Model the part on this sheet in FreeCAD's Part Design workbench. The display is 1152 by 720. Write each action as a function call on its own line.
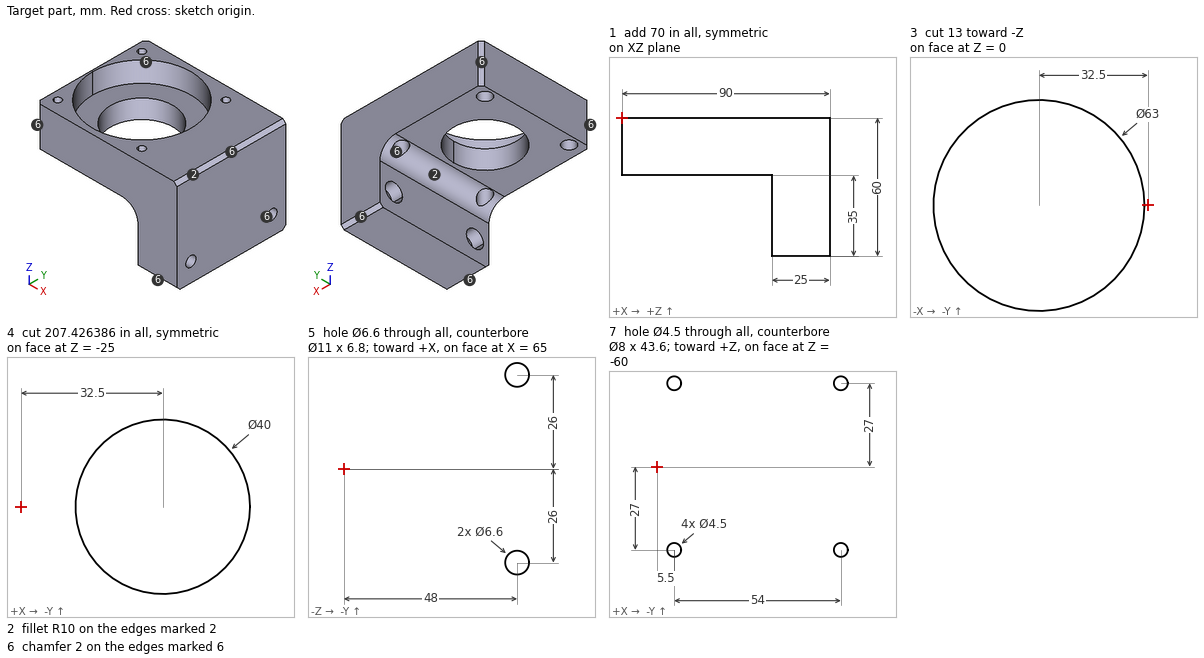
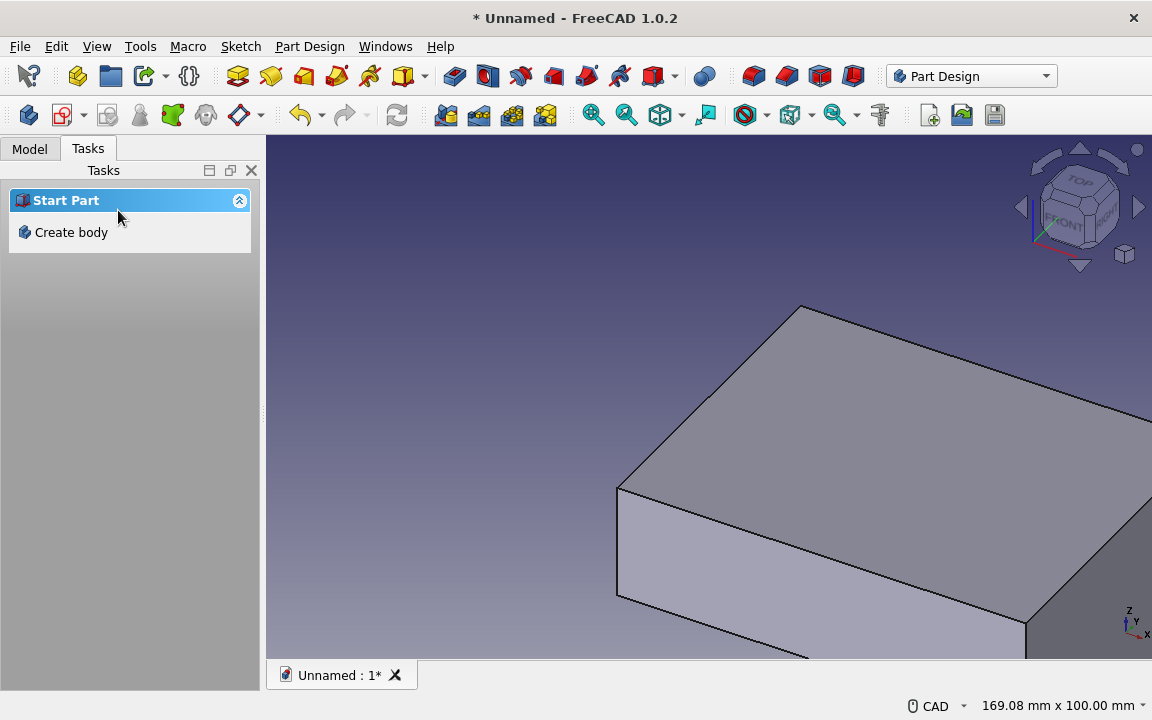
key(v)
key(f)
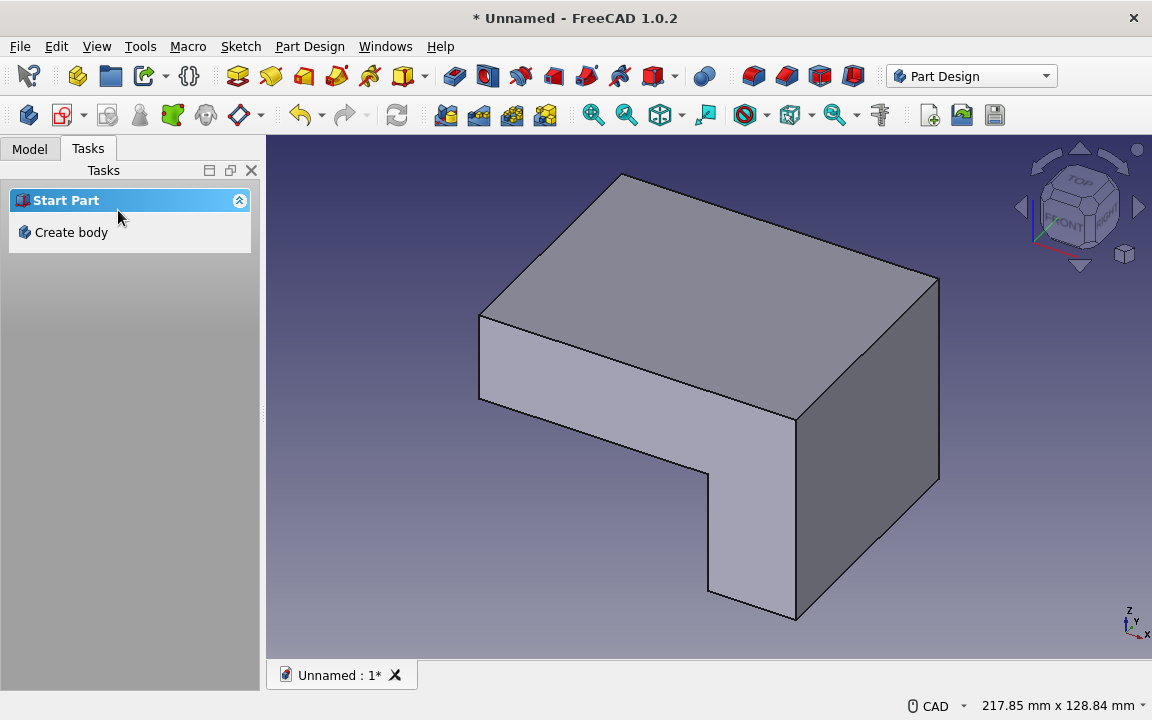
key(0)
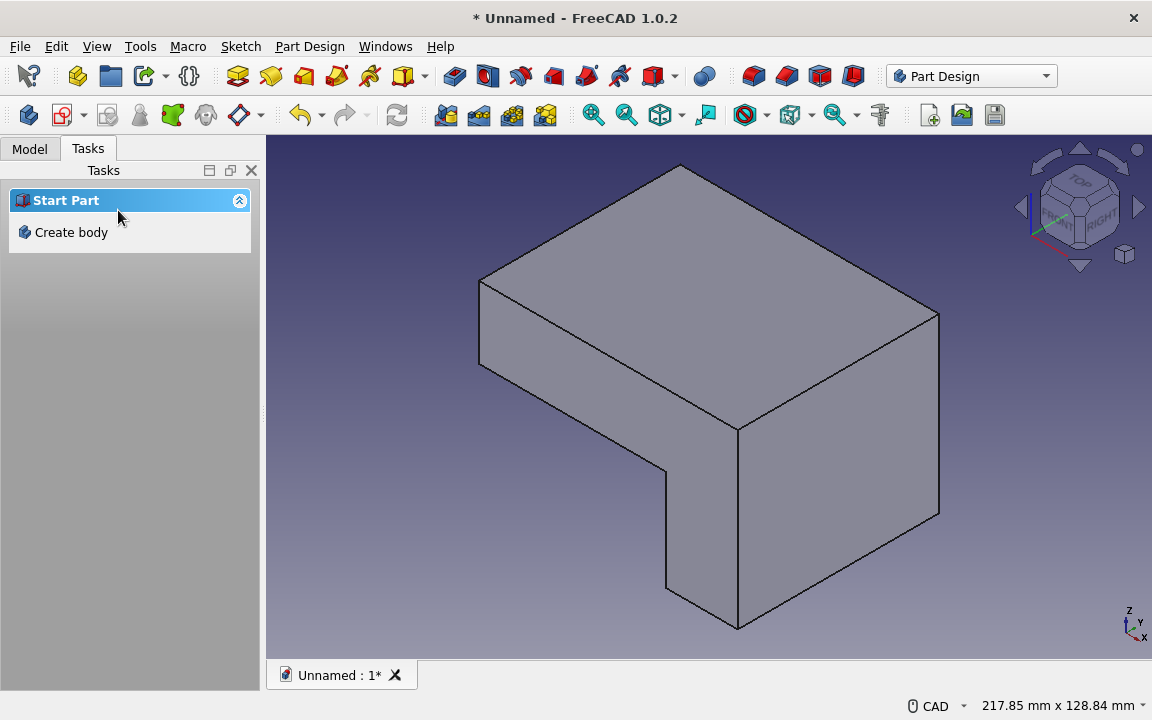
key(2)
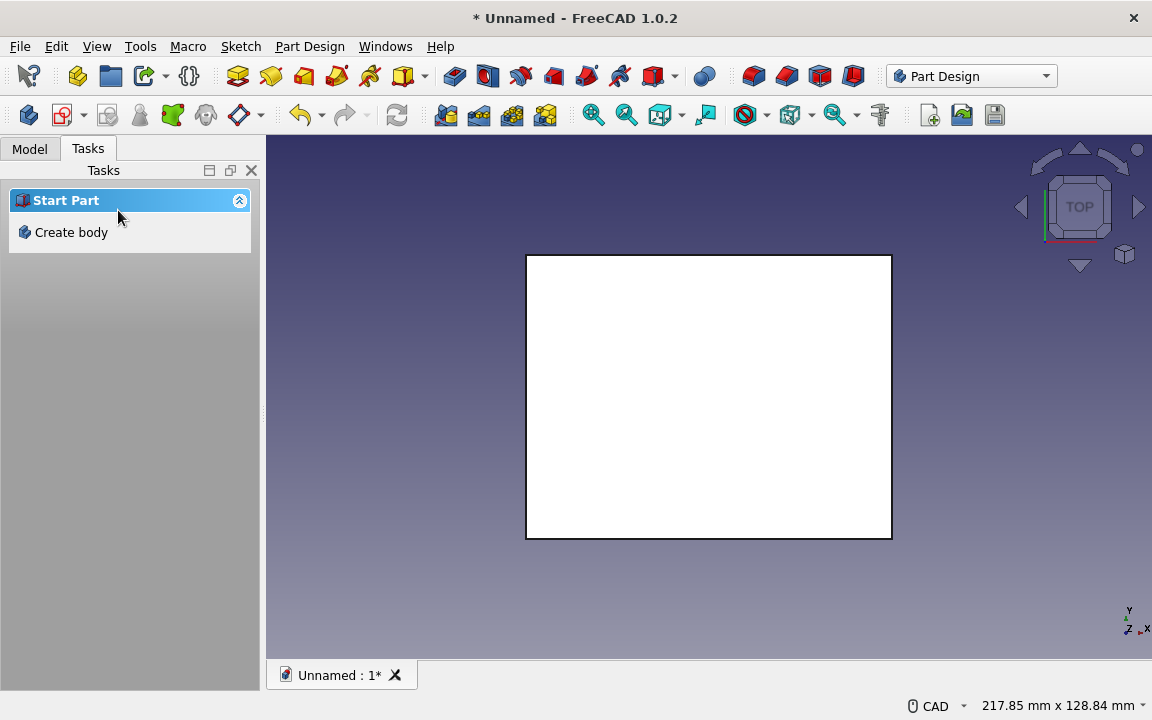
key(1)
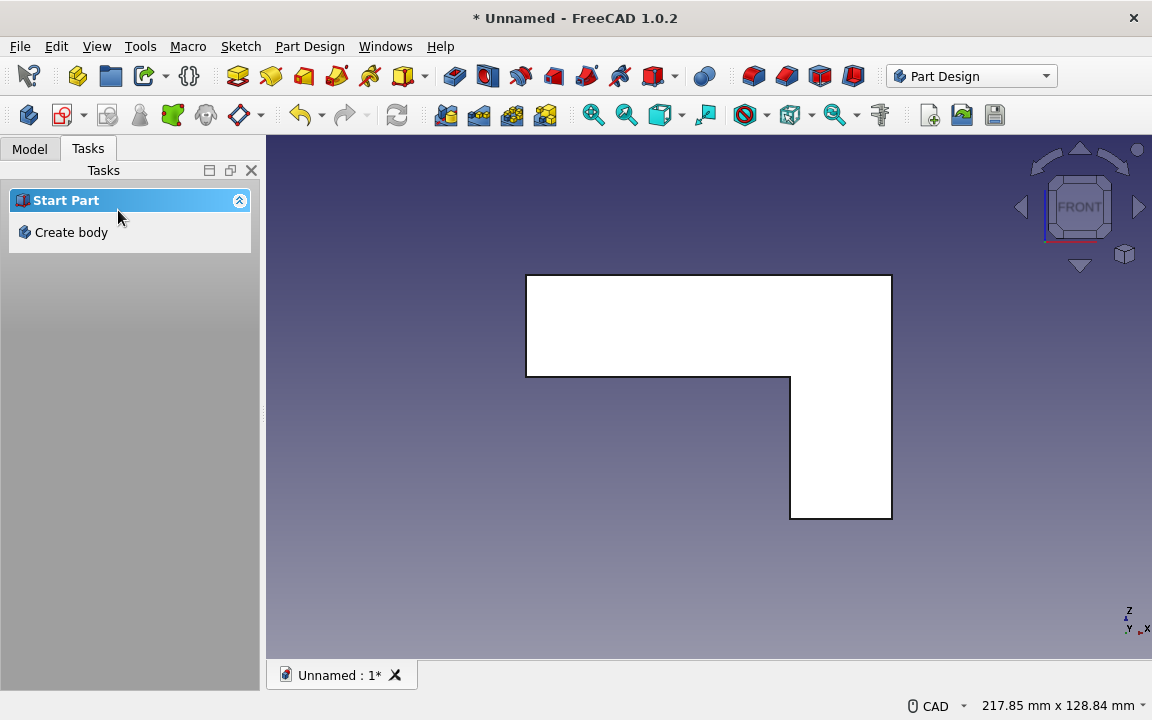
key(3)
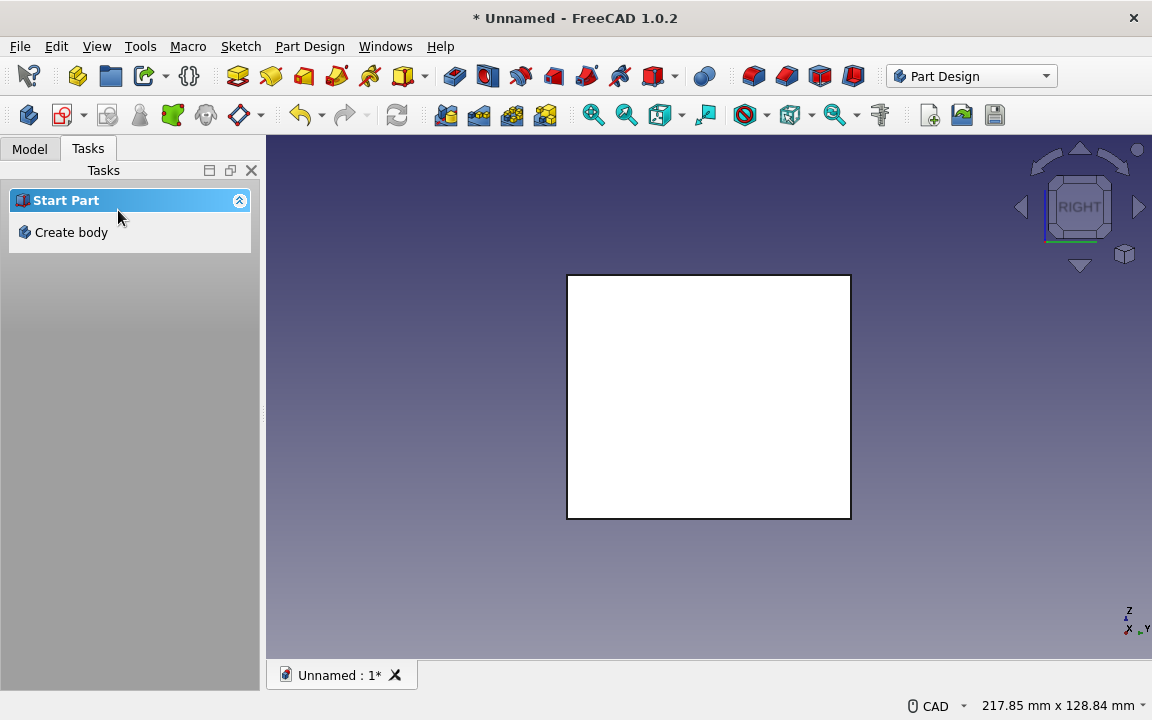
key(5)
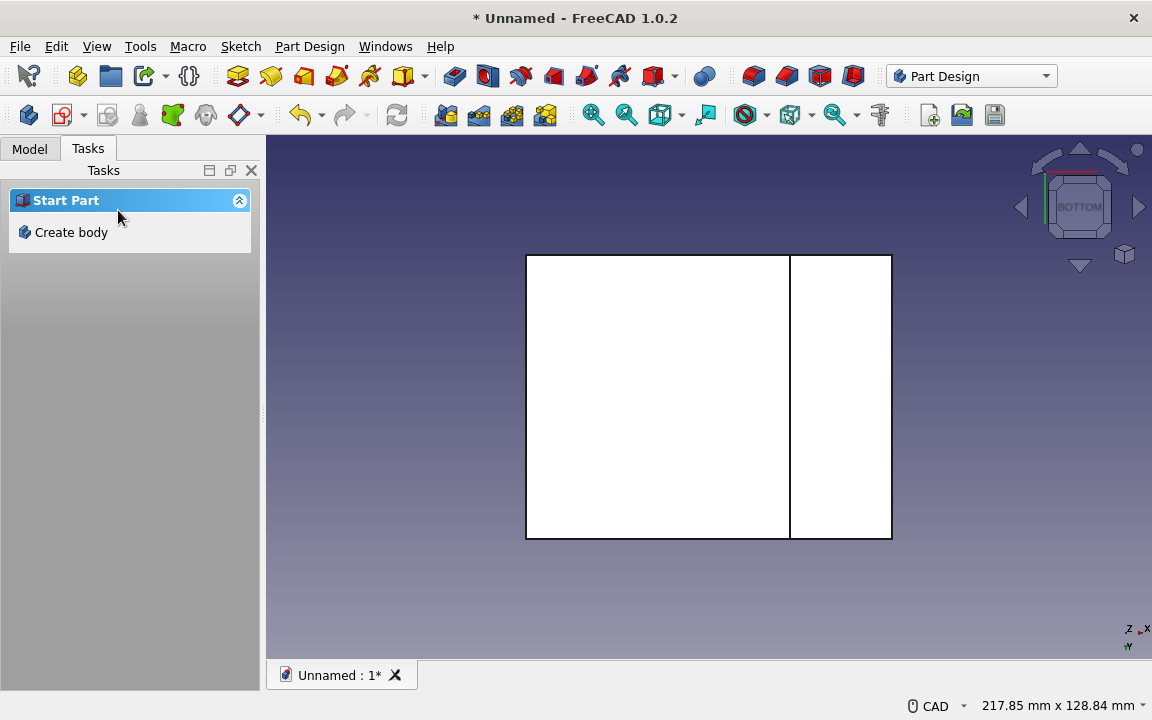
key(4)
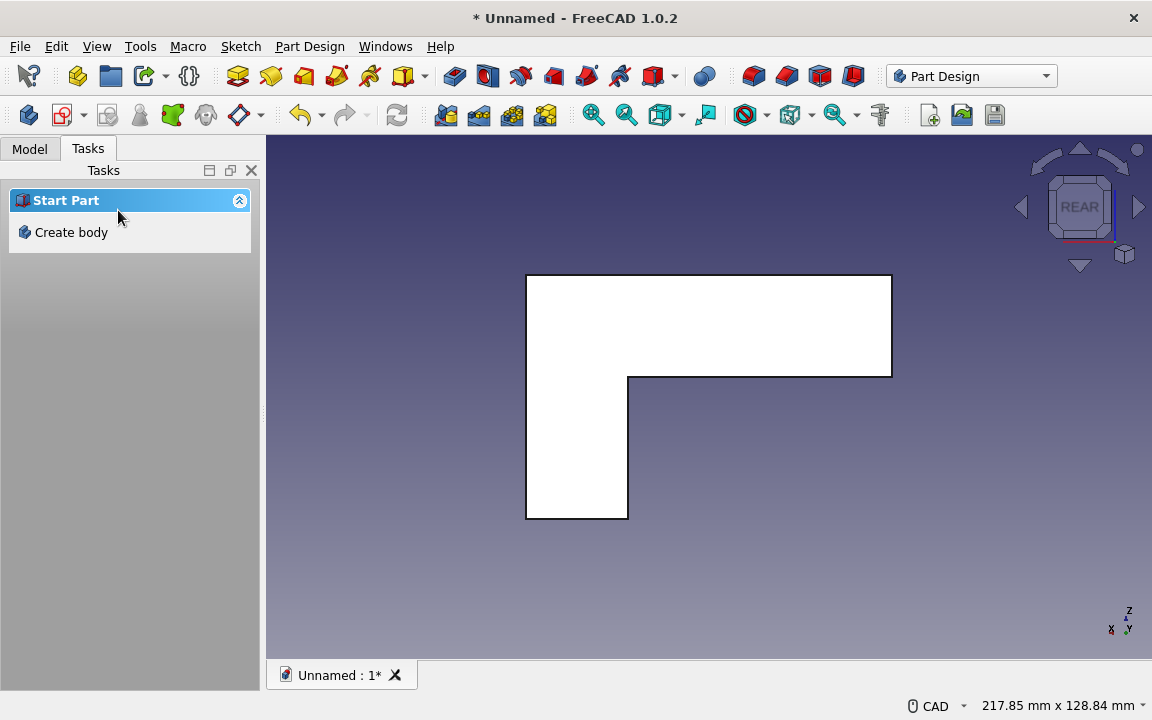
key(6)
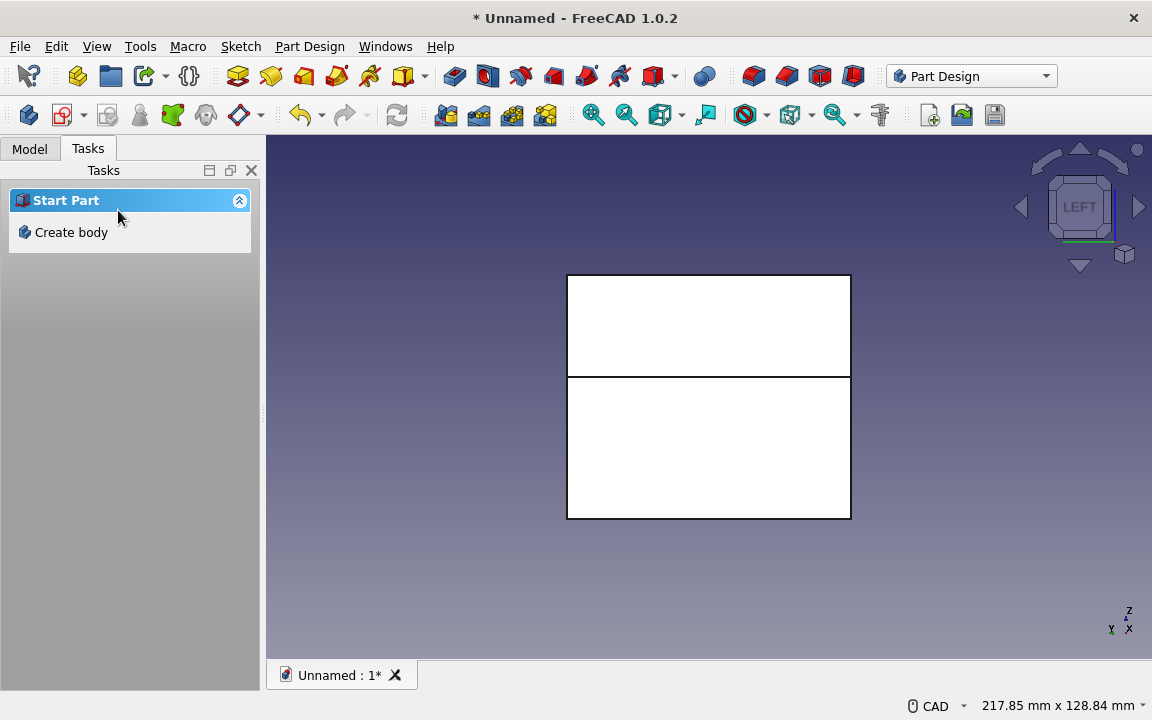
key(v)
key(3)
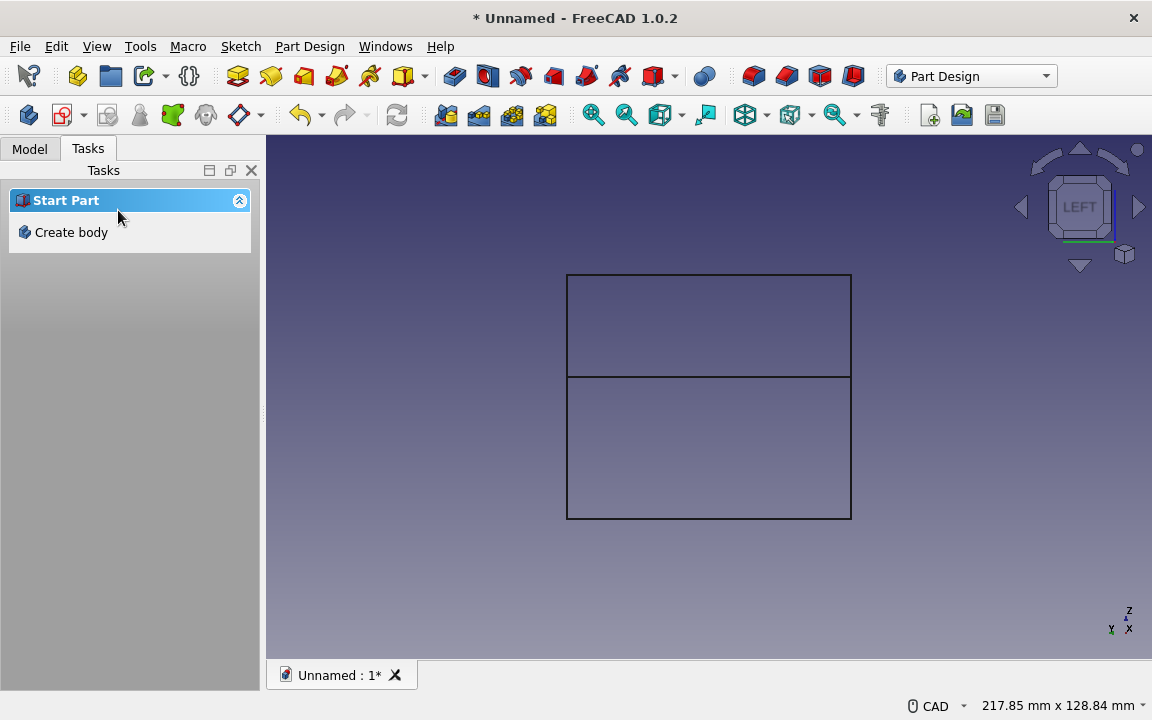
key(0)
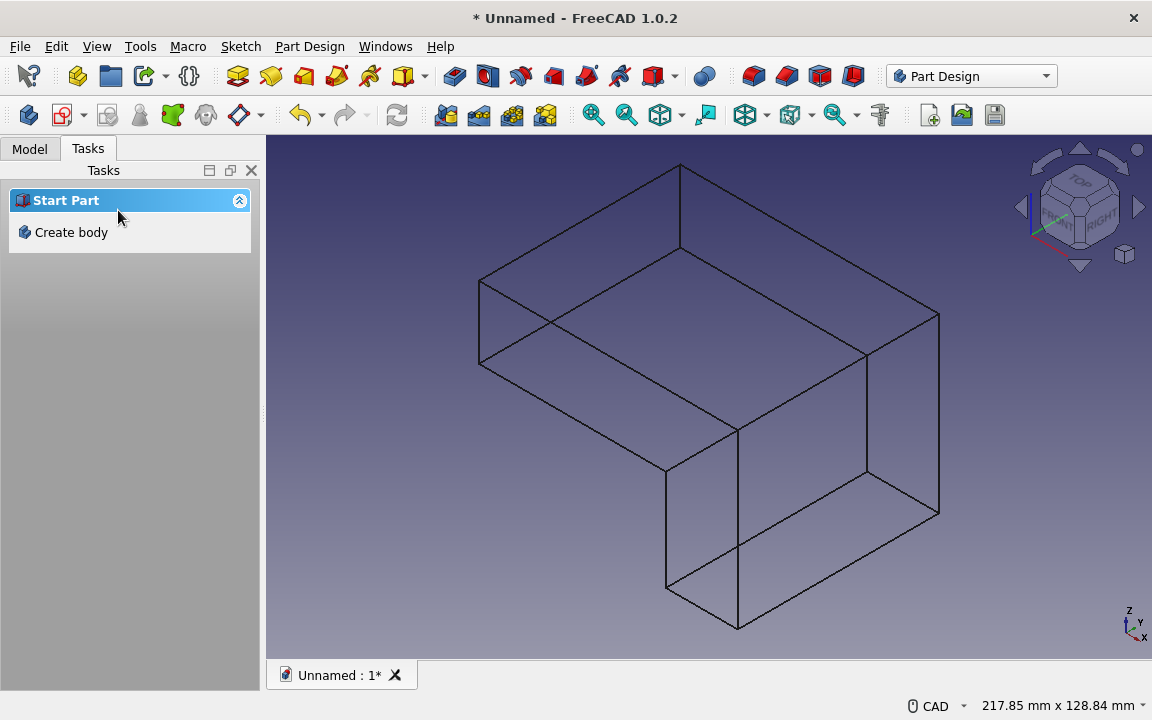
click(726, 436)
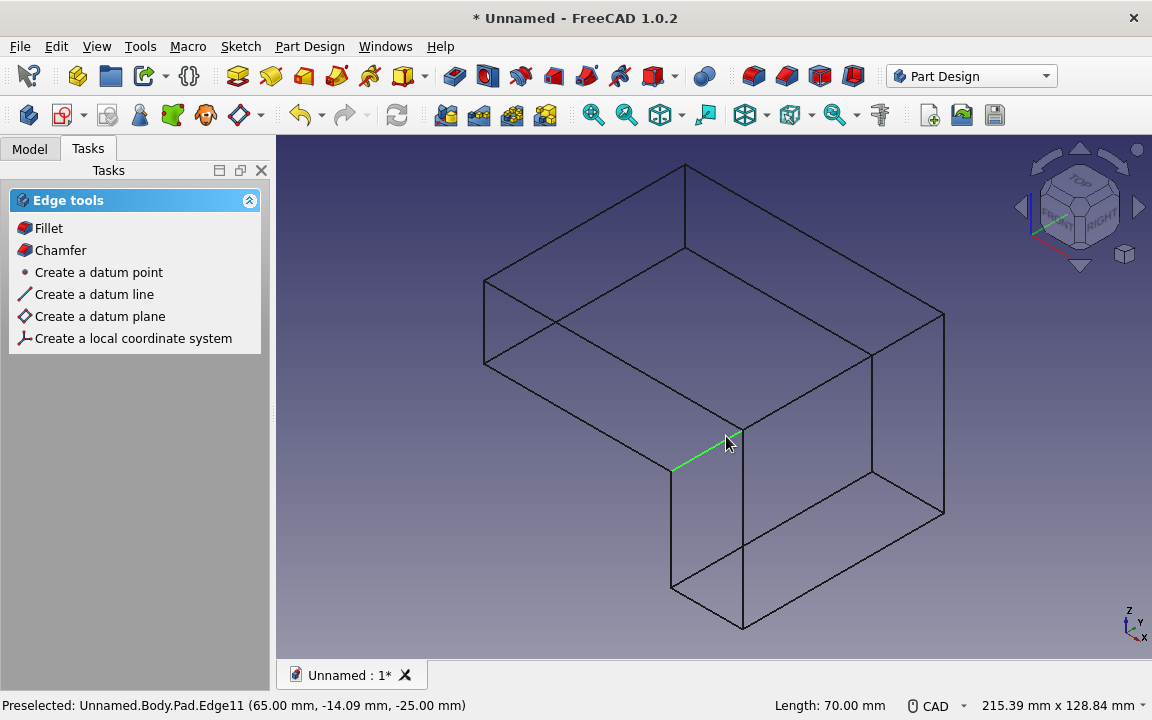
key(v)
key(1)